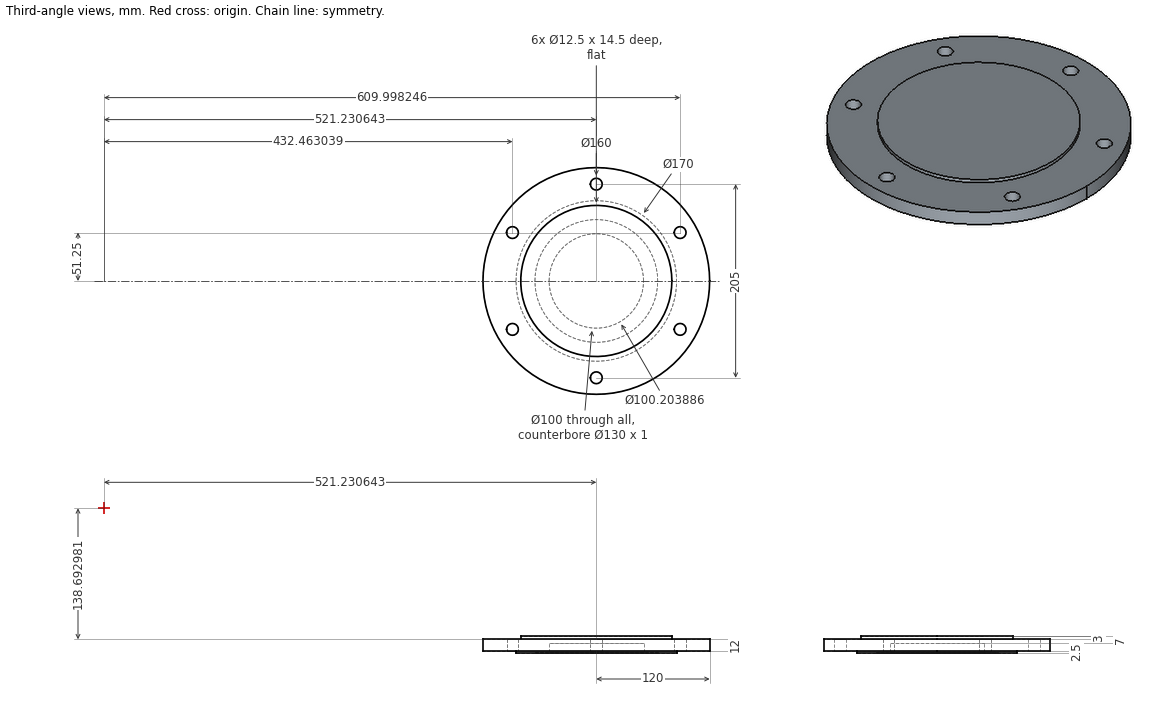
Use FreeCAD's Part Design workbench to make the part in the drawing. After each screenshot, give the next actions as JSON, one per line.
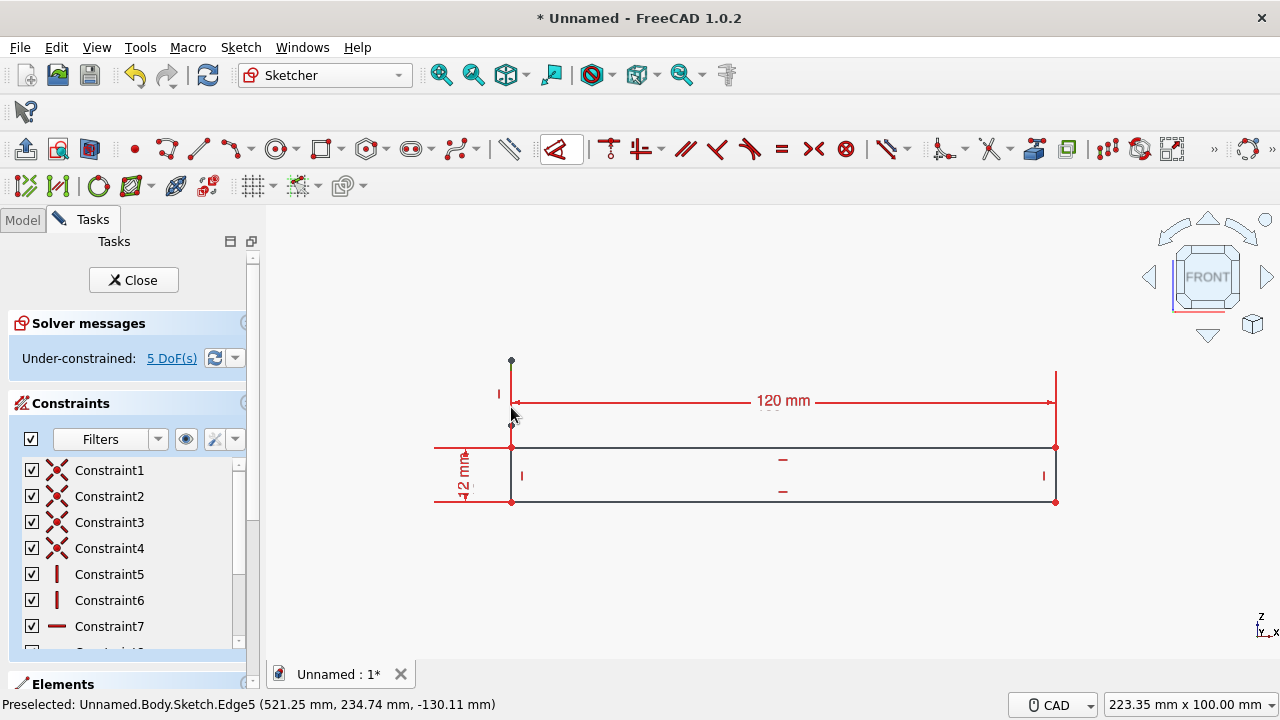
{"action": "key", "text": "g n"}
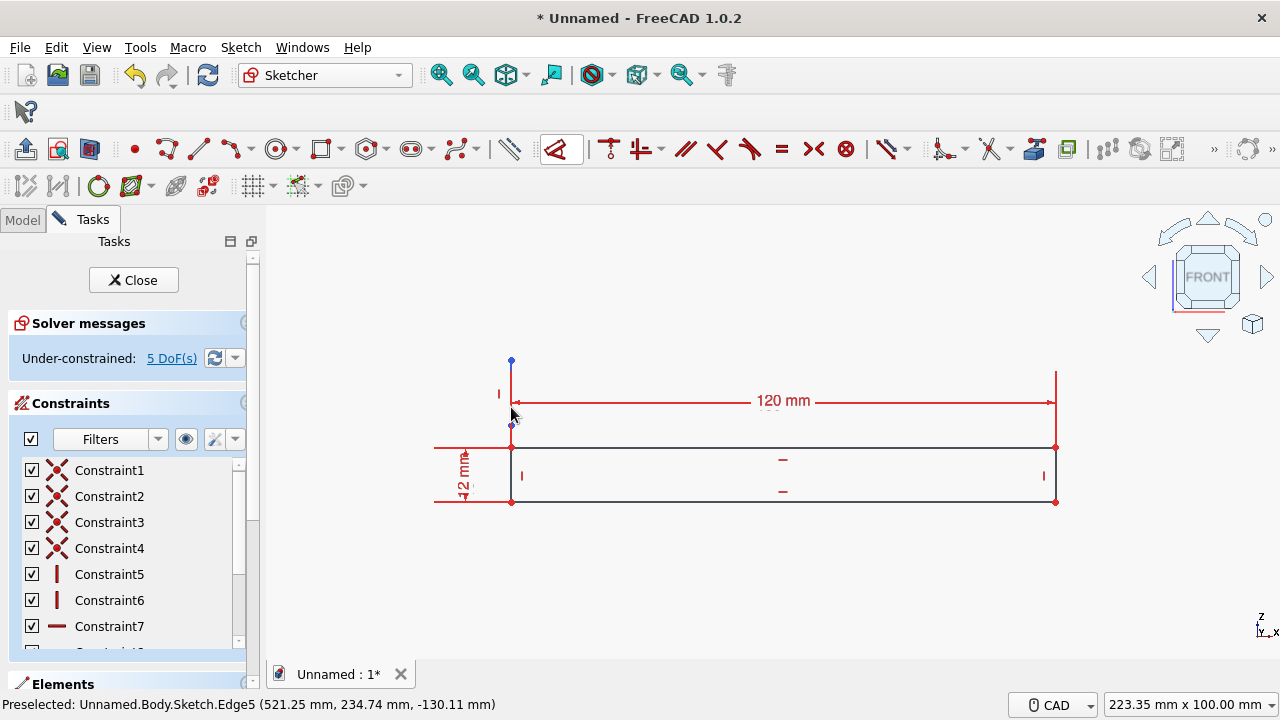
{"action": "key", "text": "d"}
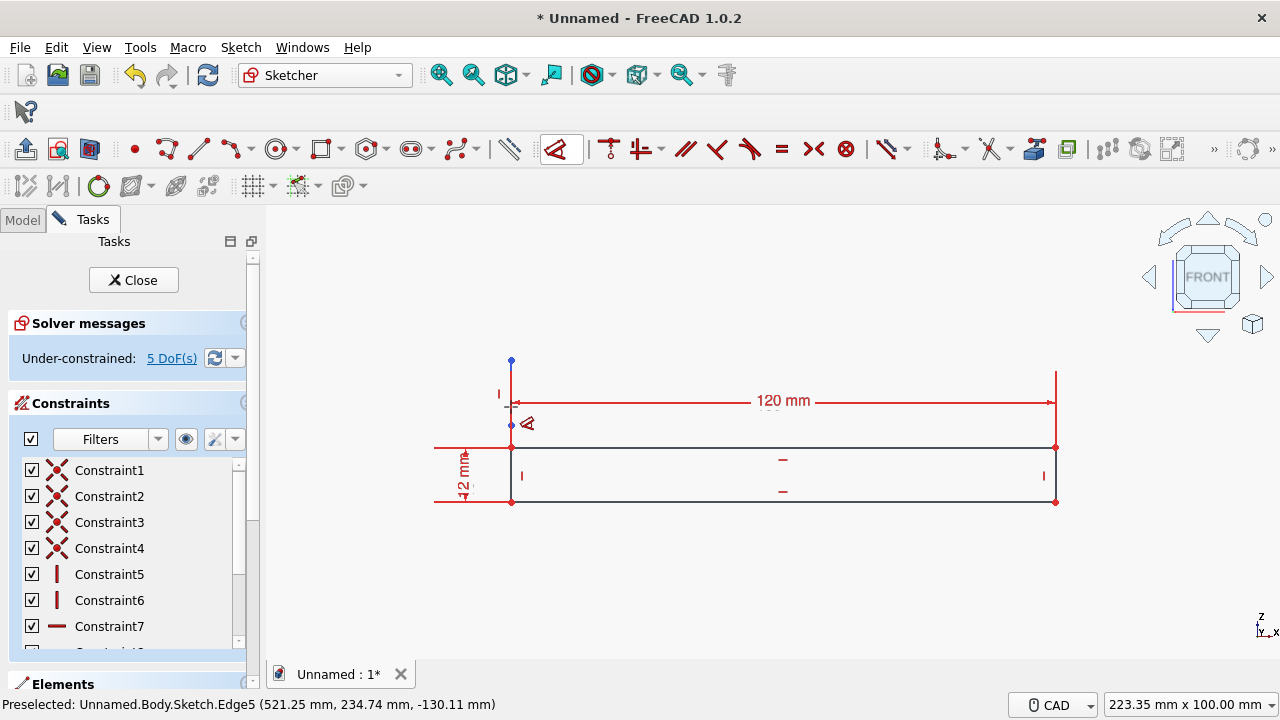
{"action": "left_click", "coordinate": [511, 448]}
{"action": "left_click", "coordinate": [403, 482]}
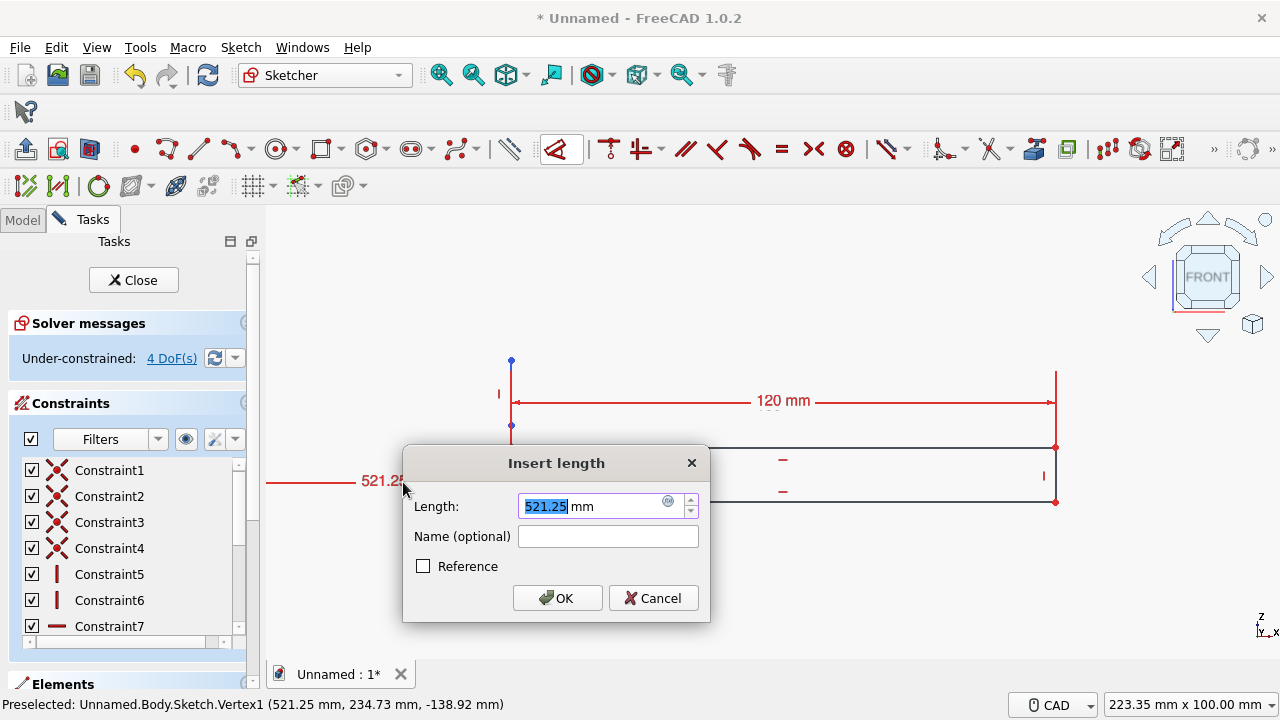
{"action": "type", "text": "521.230643"}
{"action": "key", "text": "Return"}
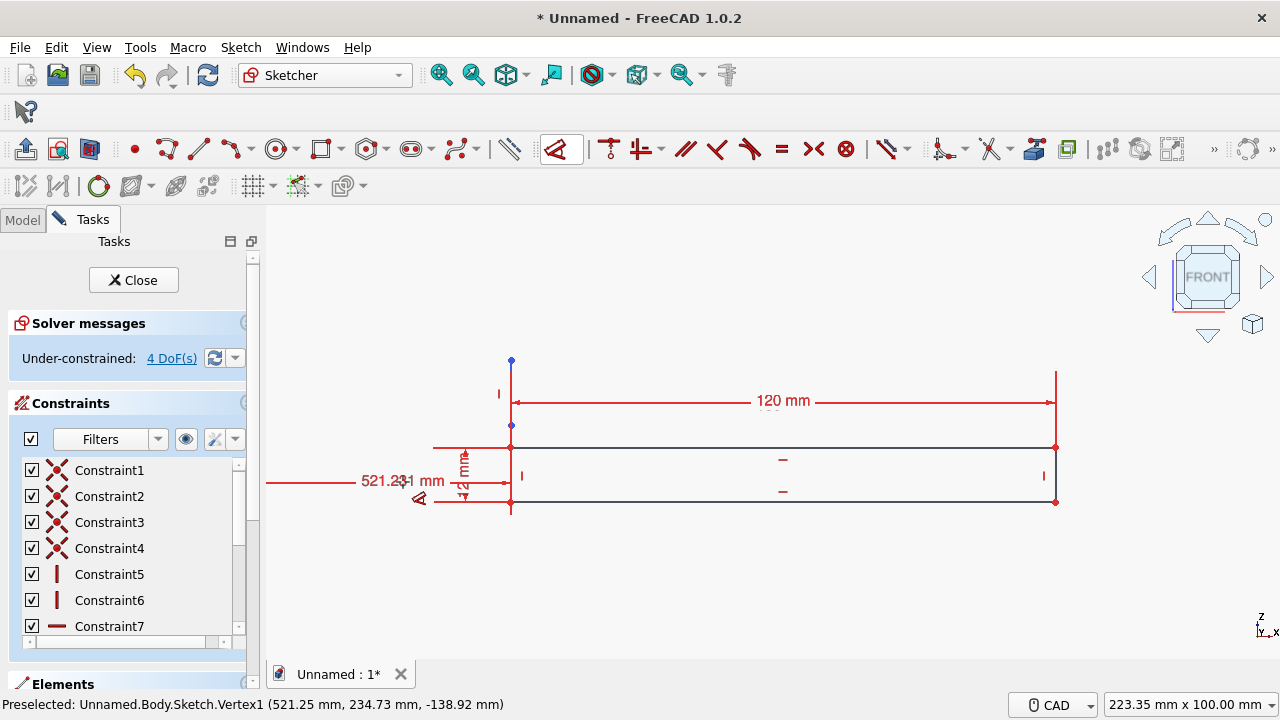
{"action": "left_click", "coordinate": [511, 448]}
{"action": "left_click", "coordinate": [545, 341]}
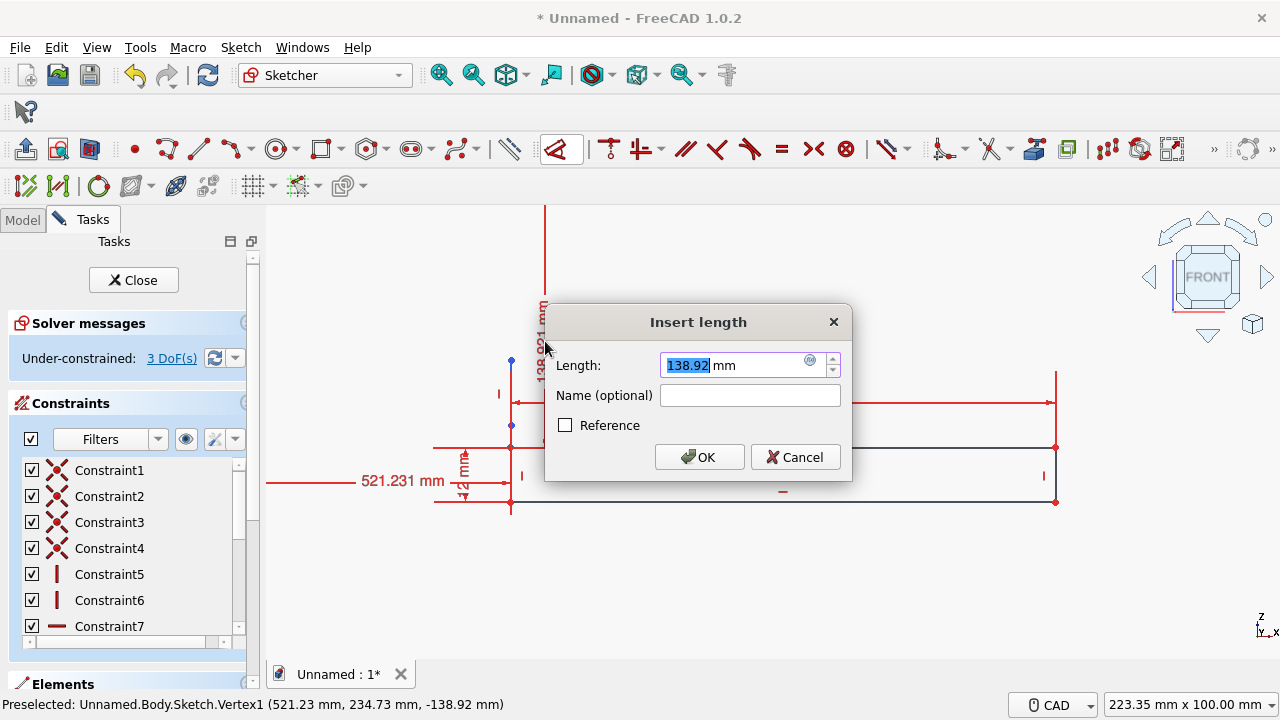
{"action": "type", "text": "138.692981"}
{"action": "key", "text": "Return"}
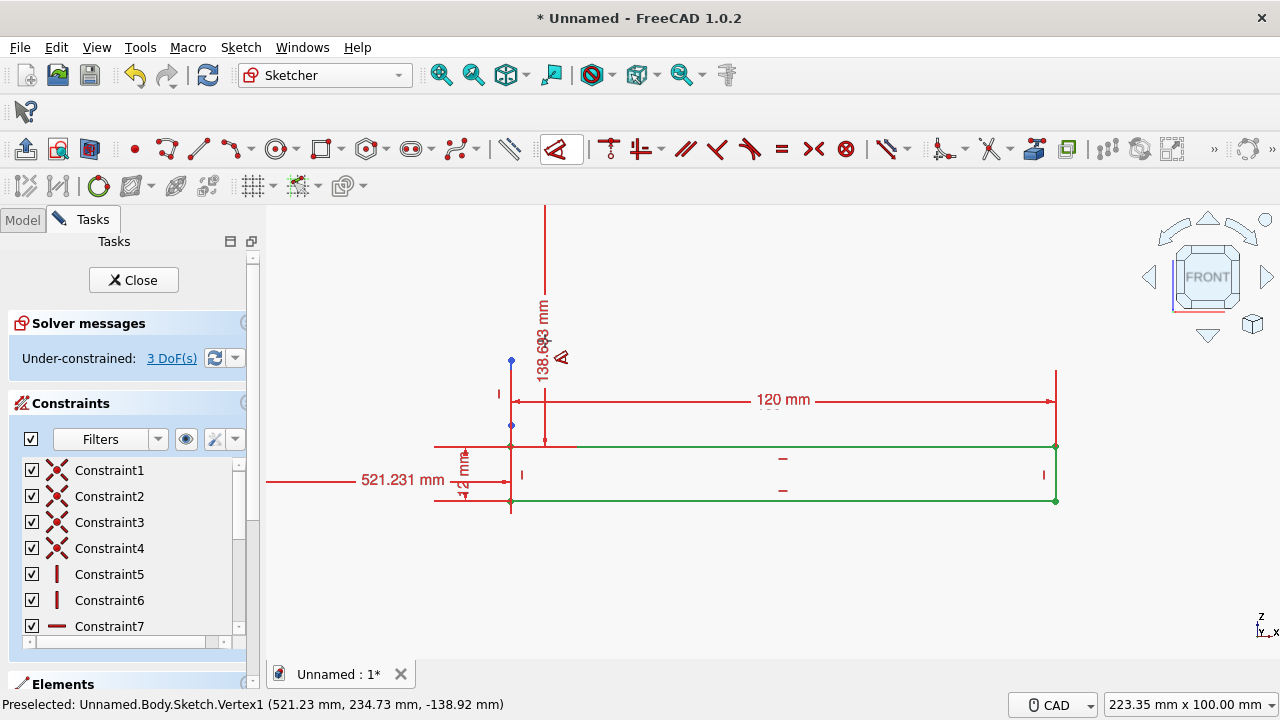
{"action": "left_click", "coordinate": [511, 426]}
{"action": "left_click", "coordinate": [403, 460]}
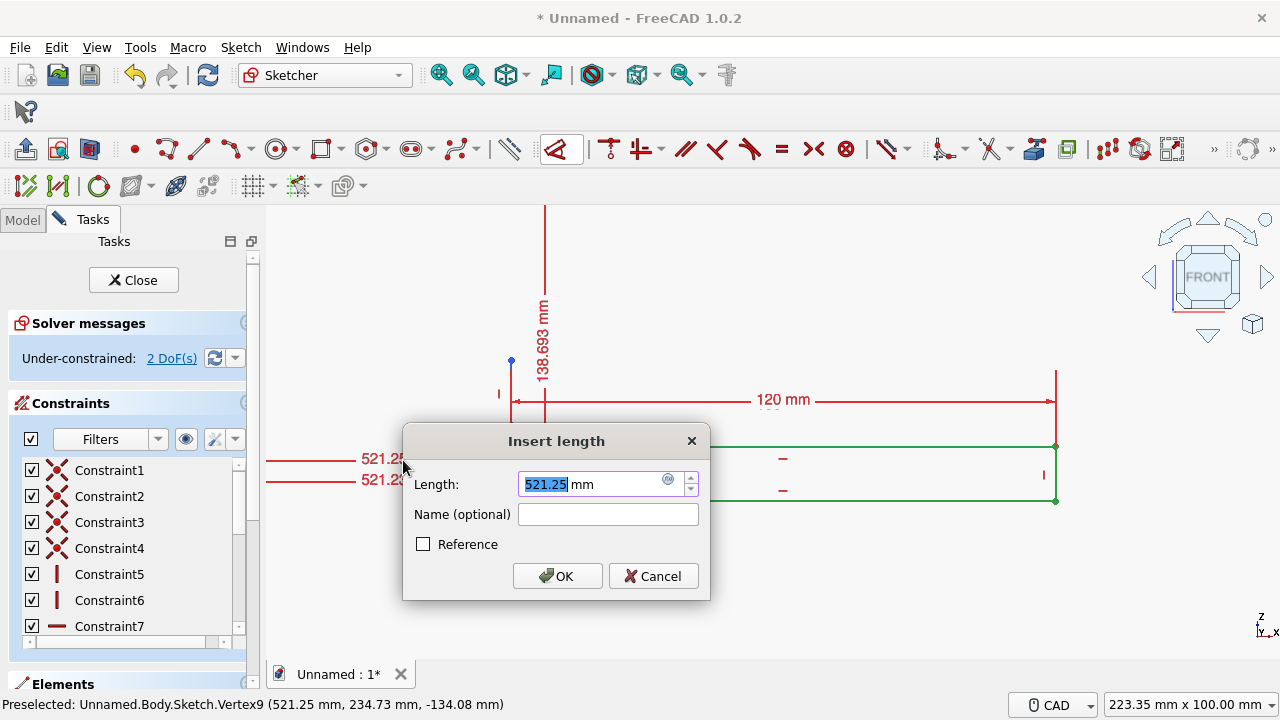
{"action": "type", "text": "521.230643"}
{"action": "key", "text": "Return"}
{"action": "key", "text": "Escape"}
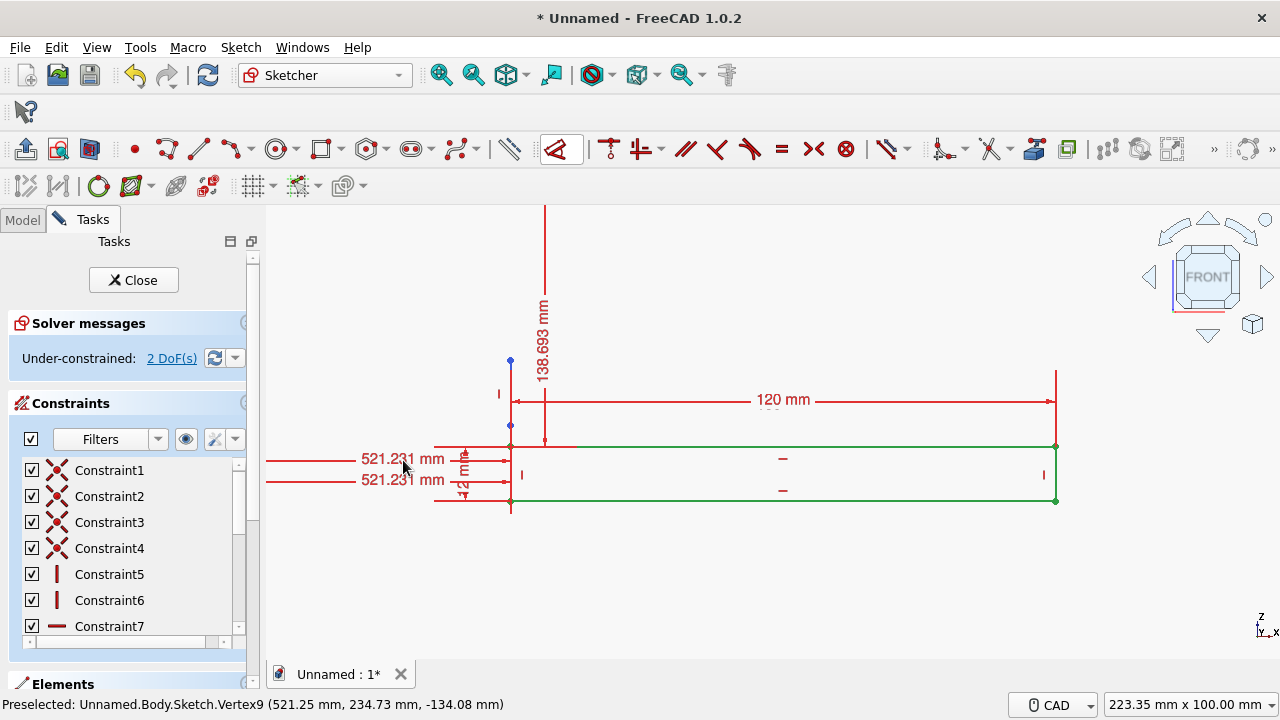
{"action": "left_click", "coordinate": [134, 280]}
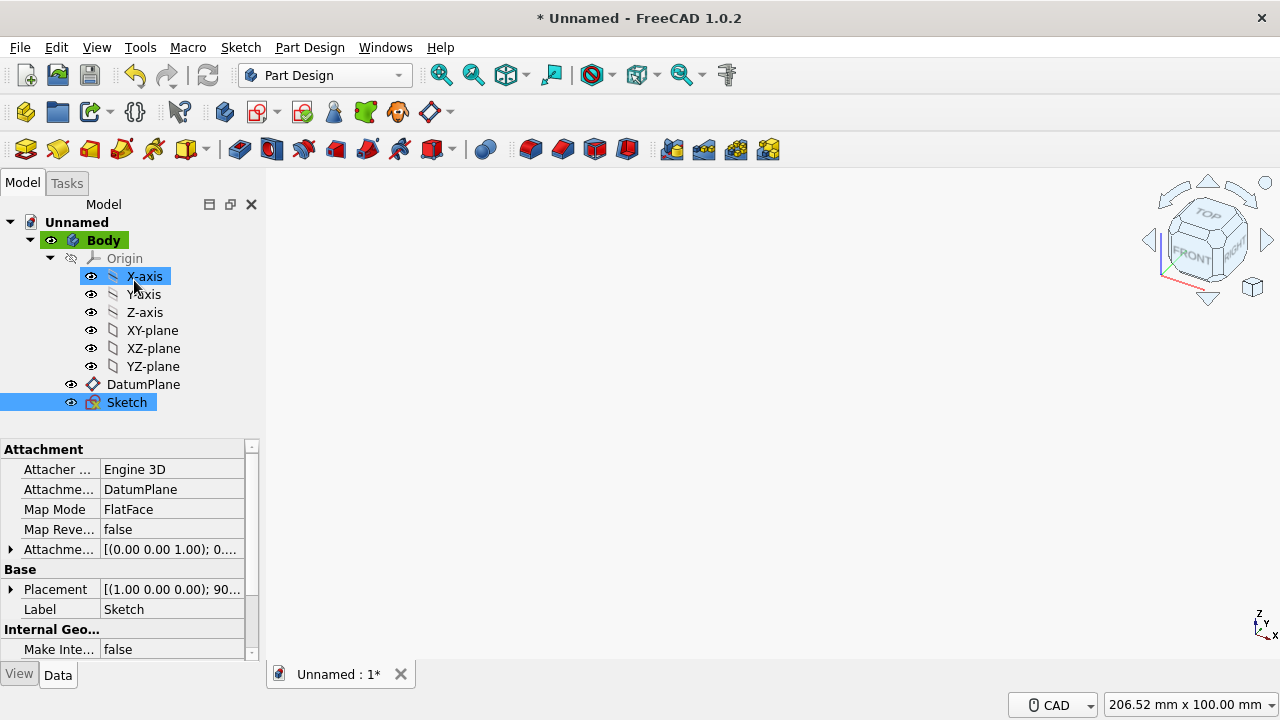
{"action": "left_click", "coordinate": [58, 150]}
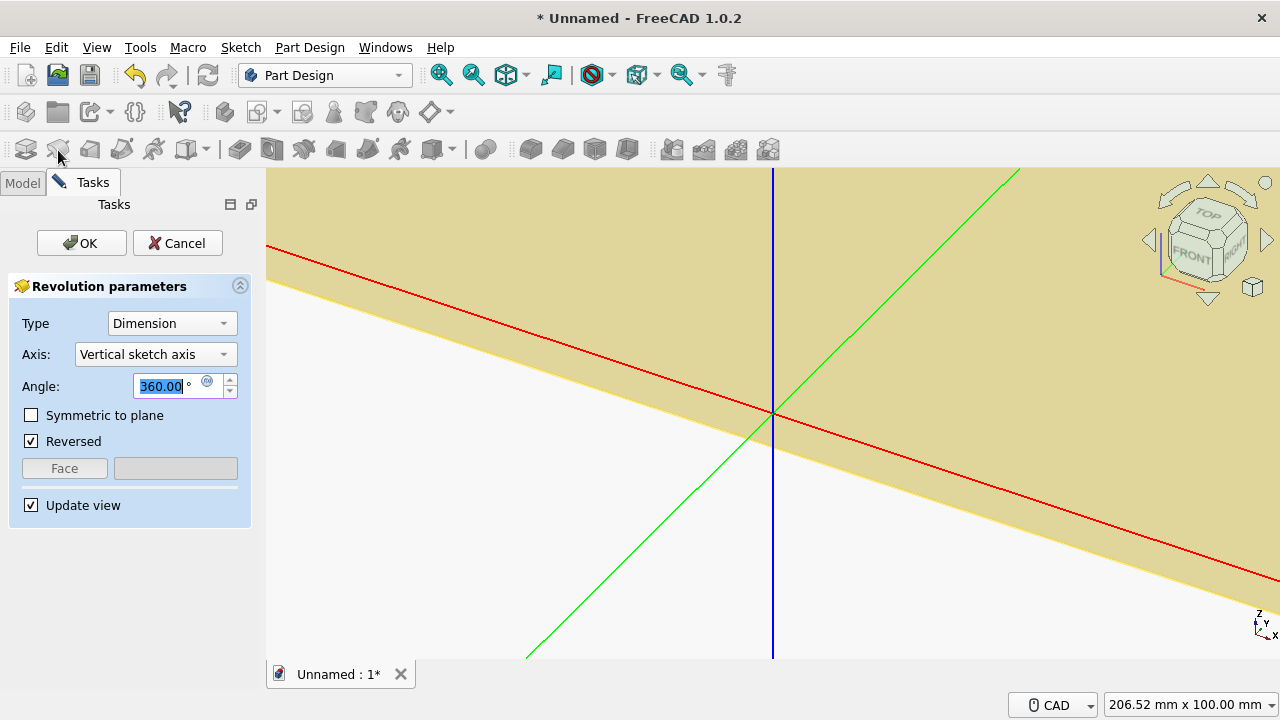
{"action": "left_click", "coordinate": [156, 354]}